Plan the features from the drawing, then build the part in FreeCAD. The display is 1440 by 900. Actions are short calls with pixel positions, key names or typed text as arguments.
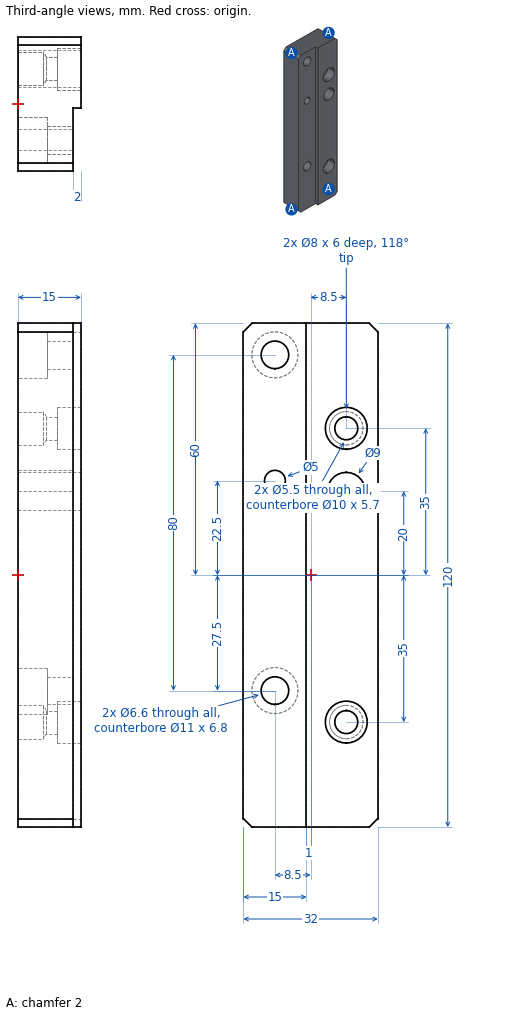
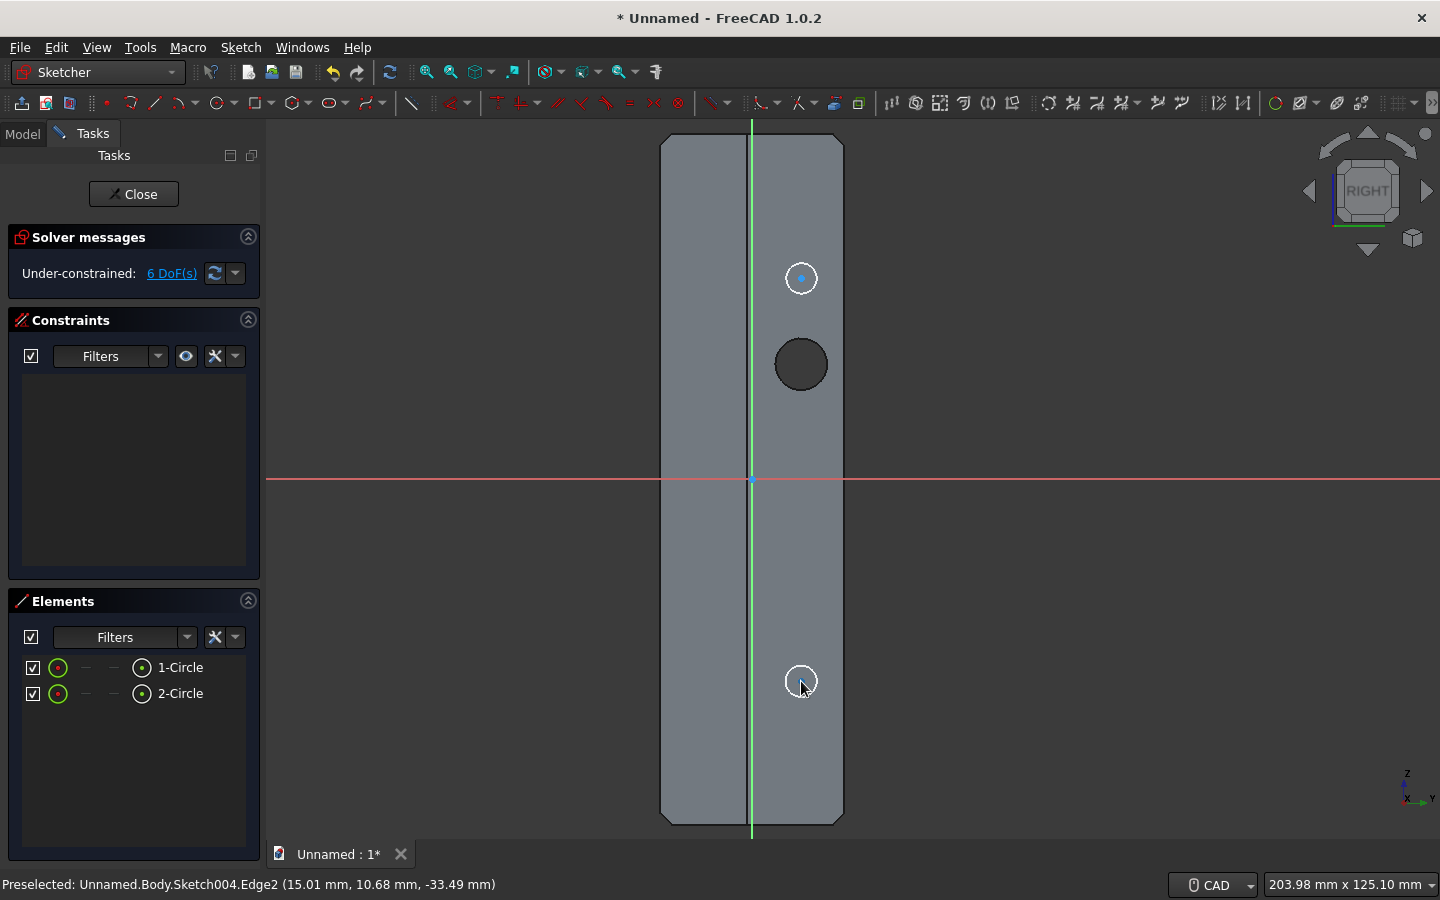
click(812, 268)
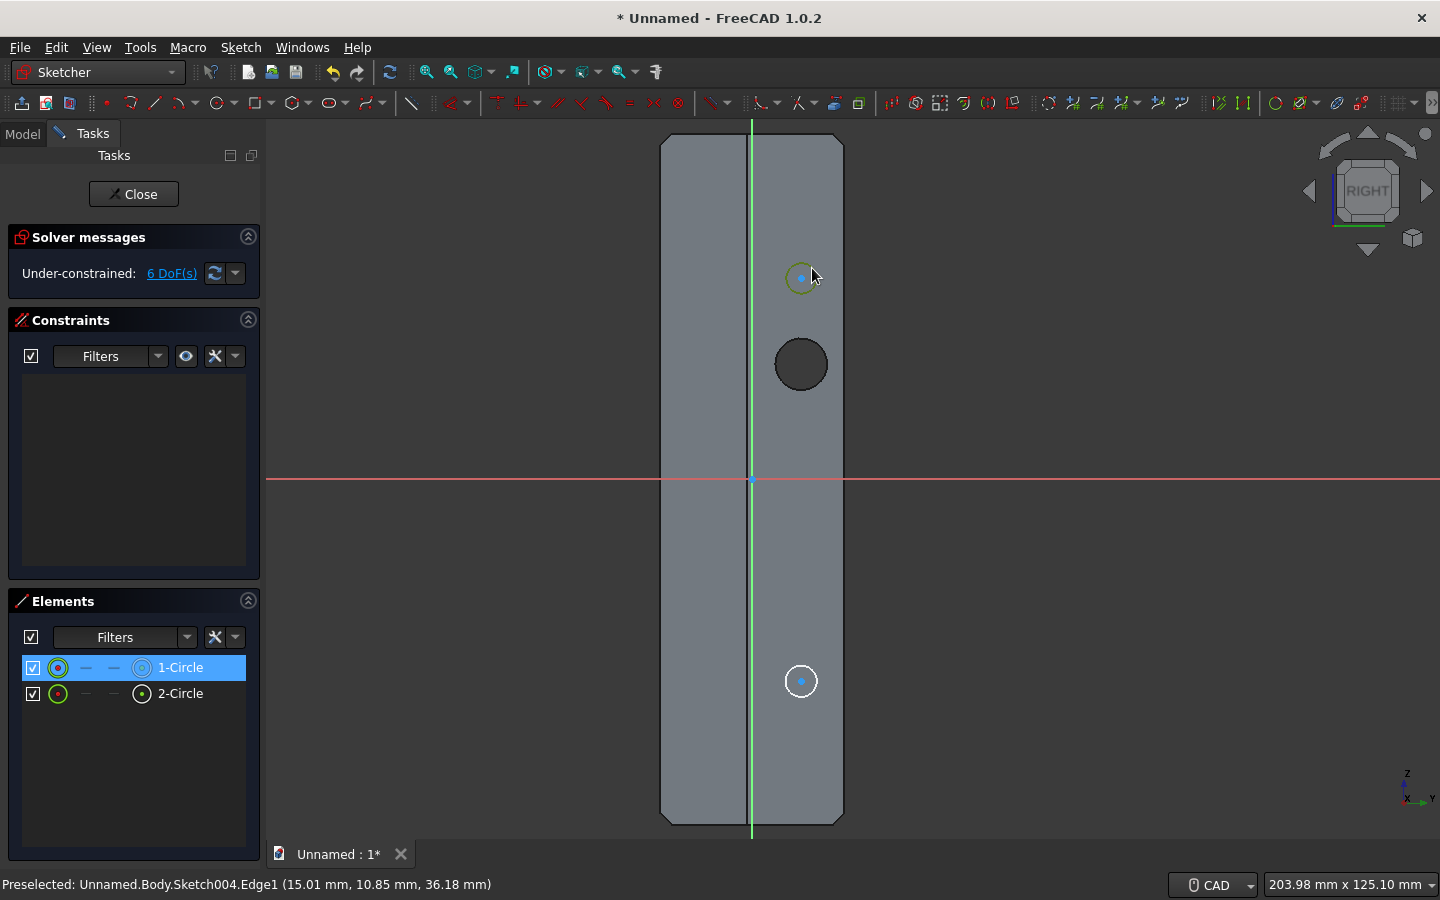
click(812, 670)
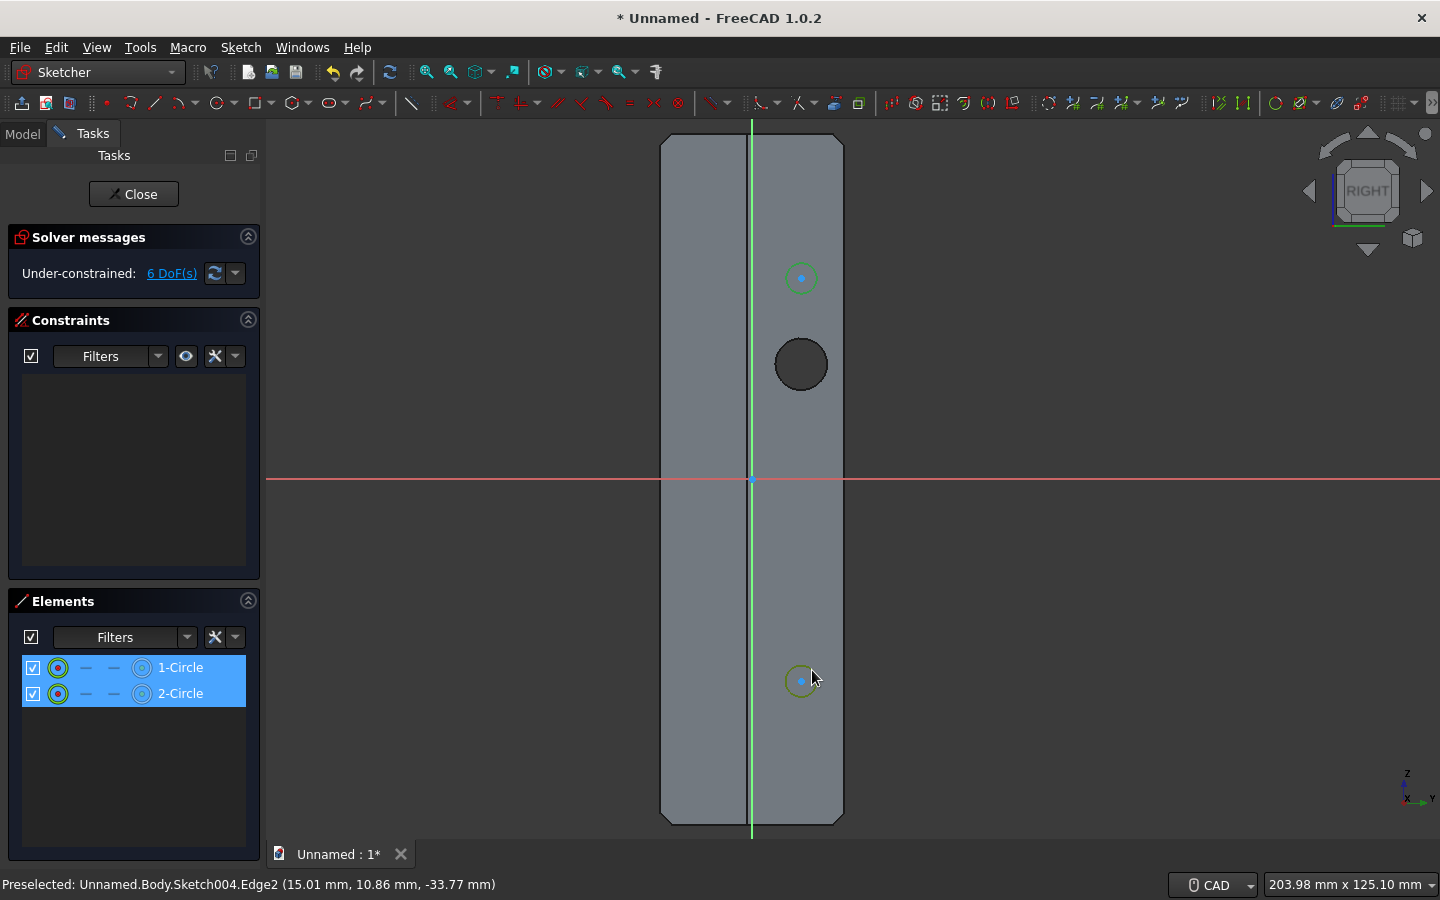
click(630, 104)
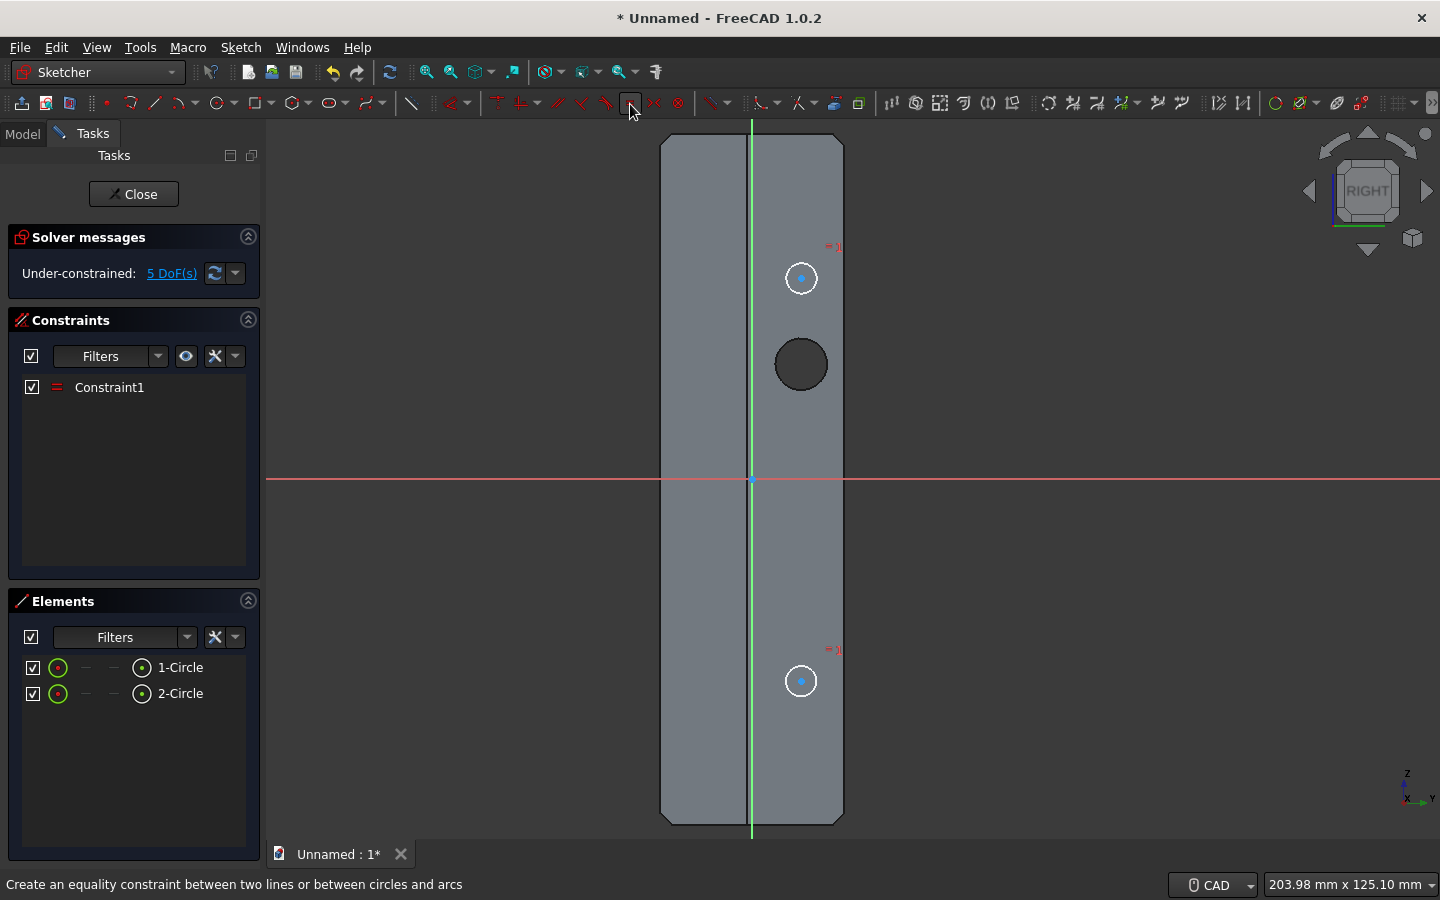
click(802, 278)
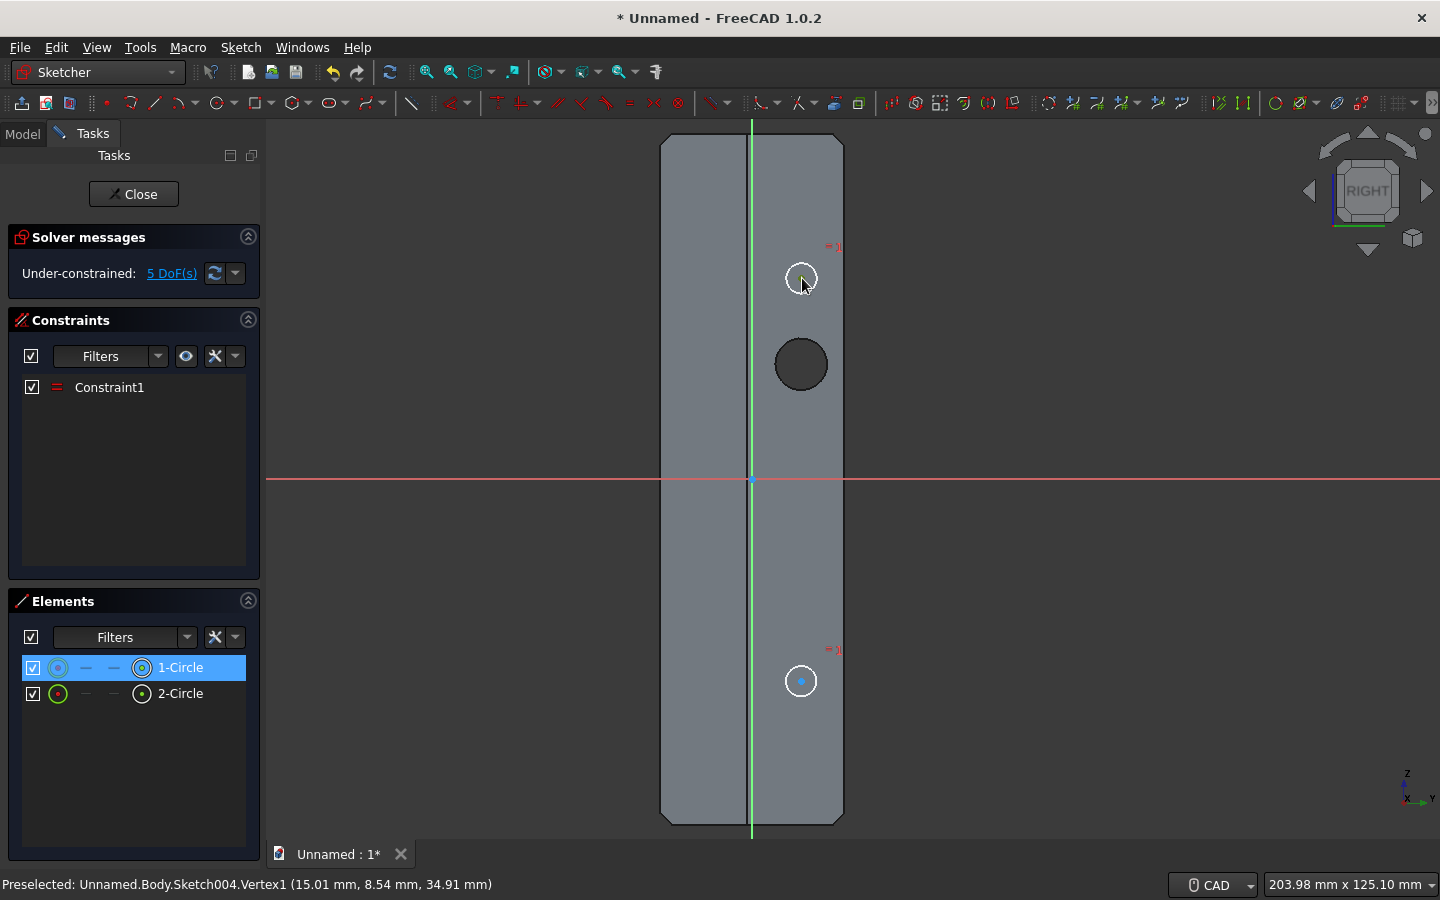
click(801, 681)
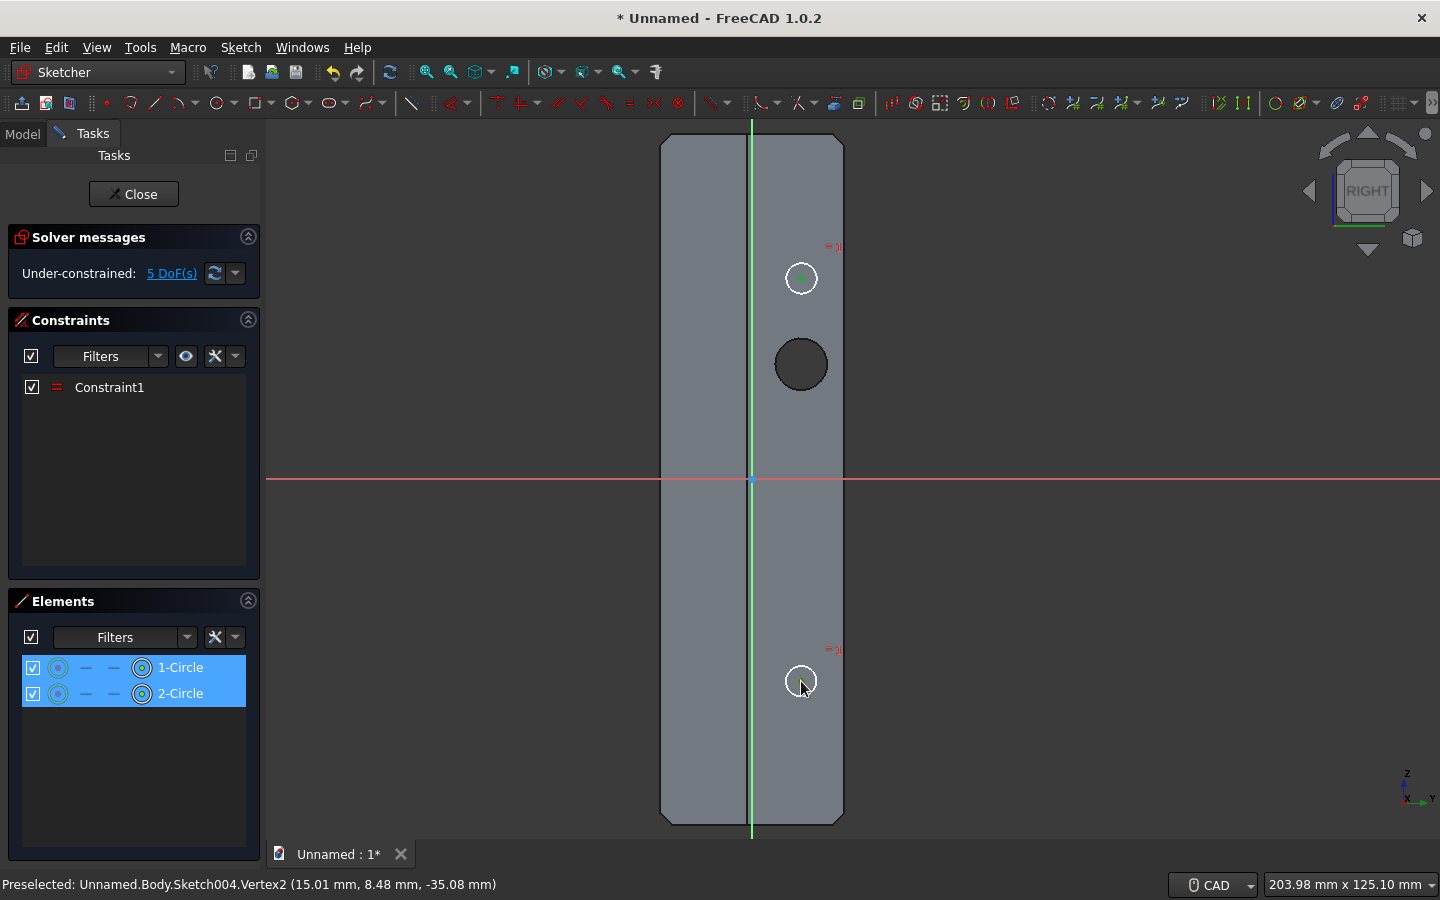
click(540, 104)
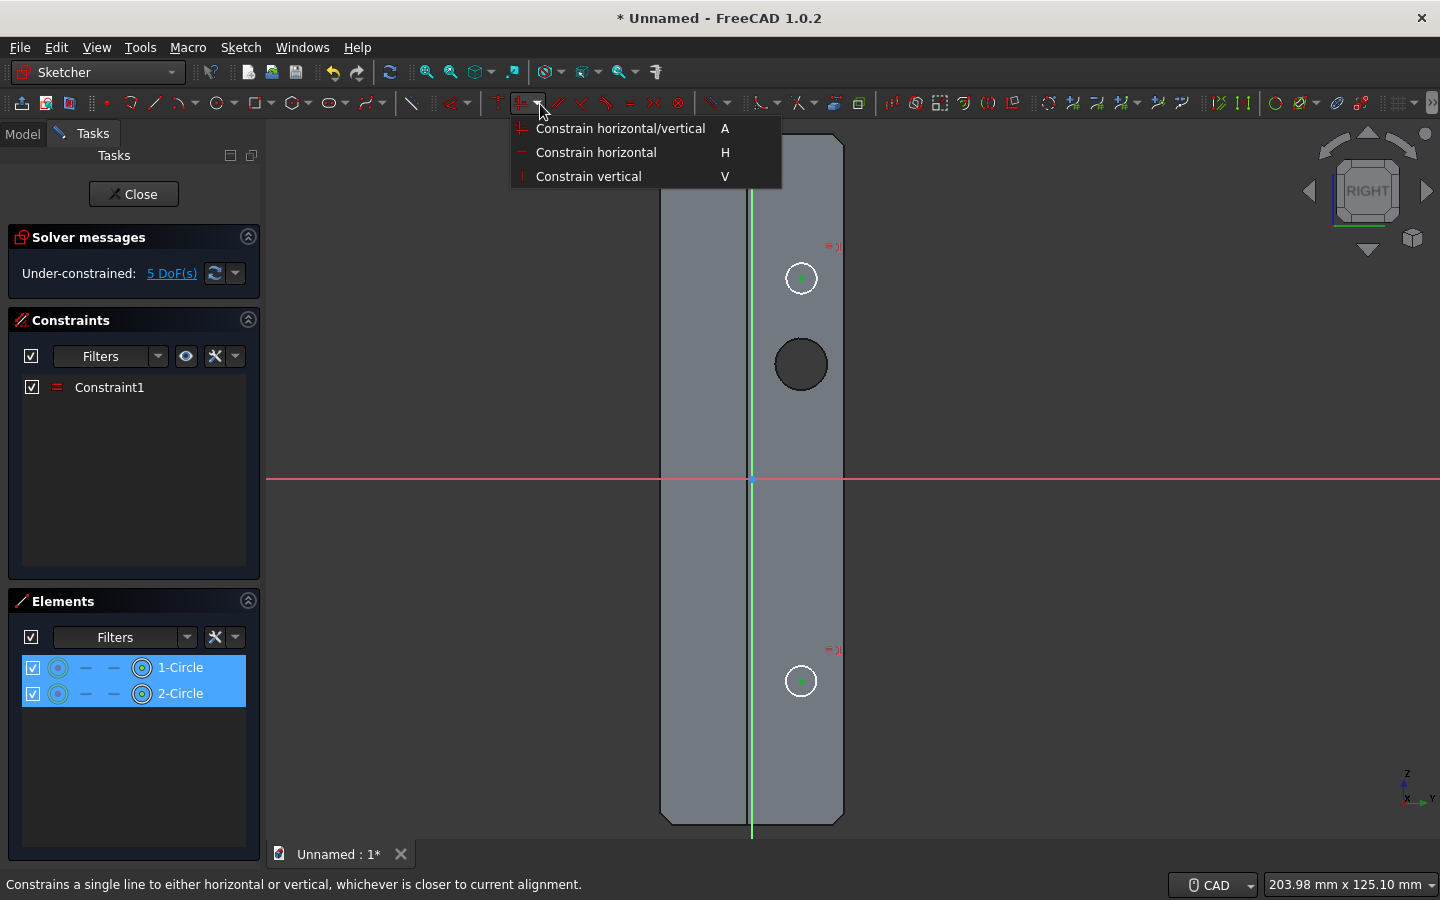
click(646, 176)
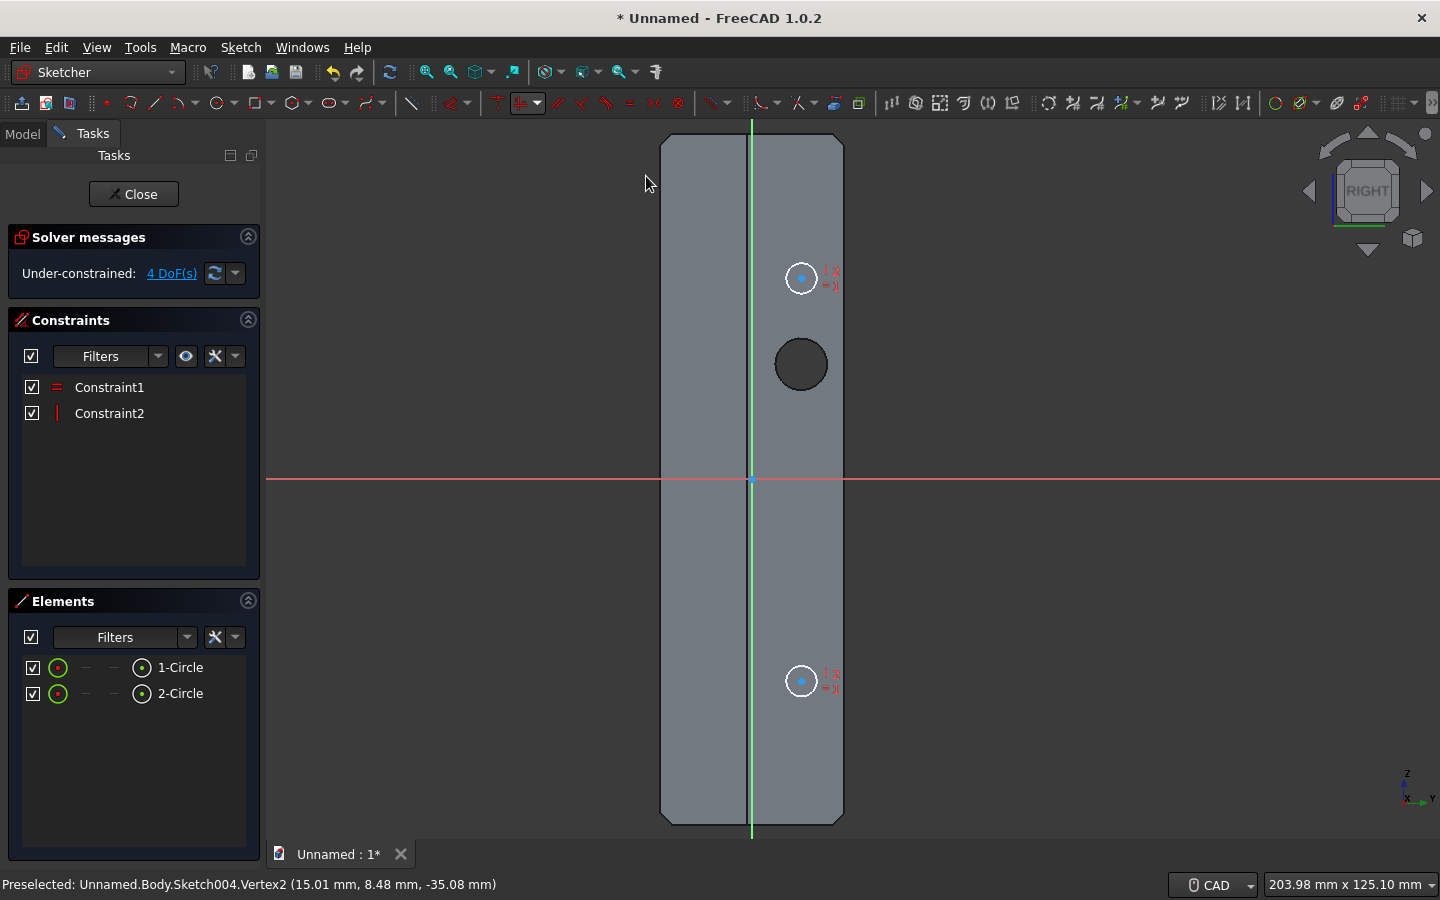
click(450, 104)